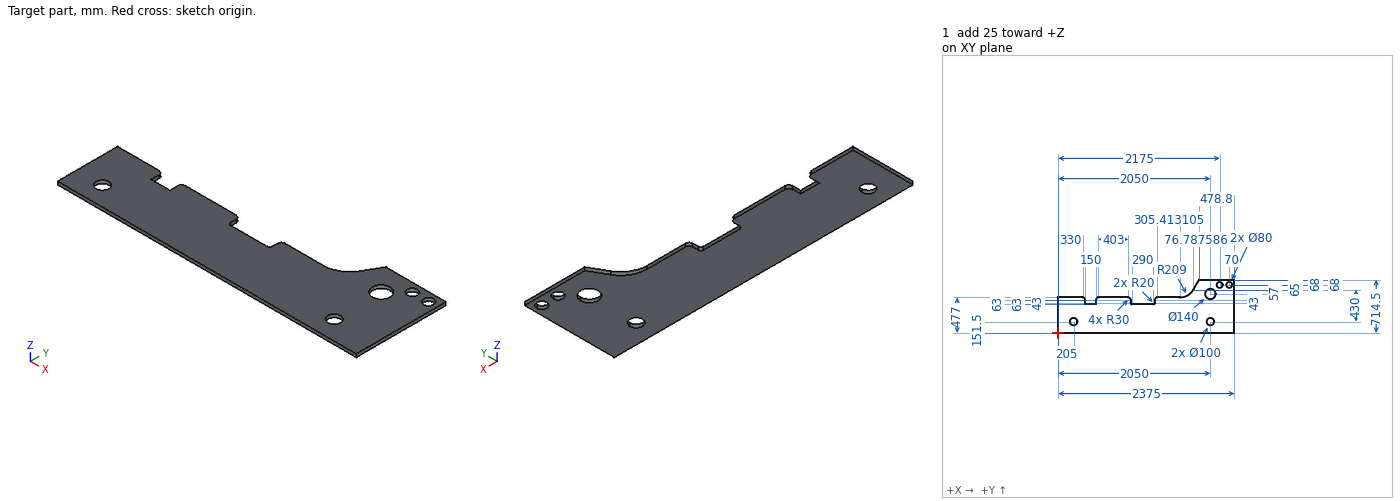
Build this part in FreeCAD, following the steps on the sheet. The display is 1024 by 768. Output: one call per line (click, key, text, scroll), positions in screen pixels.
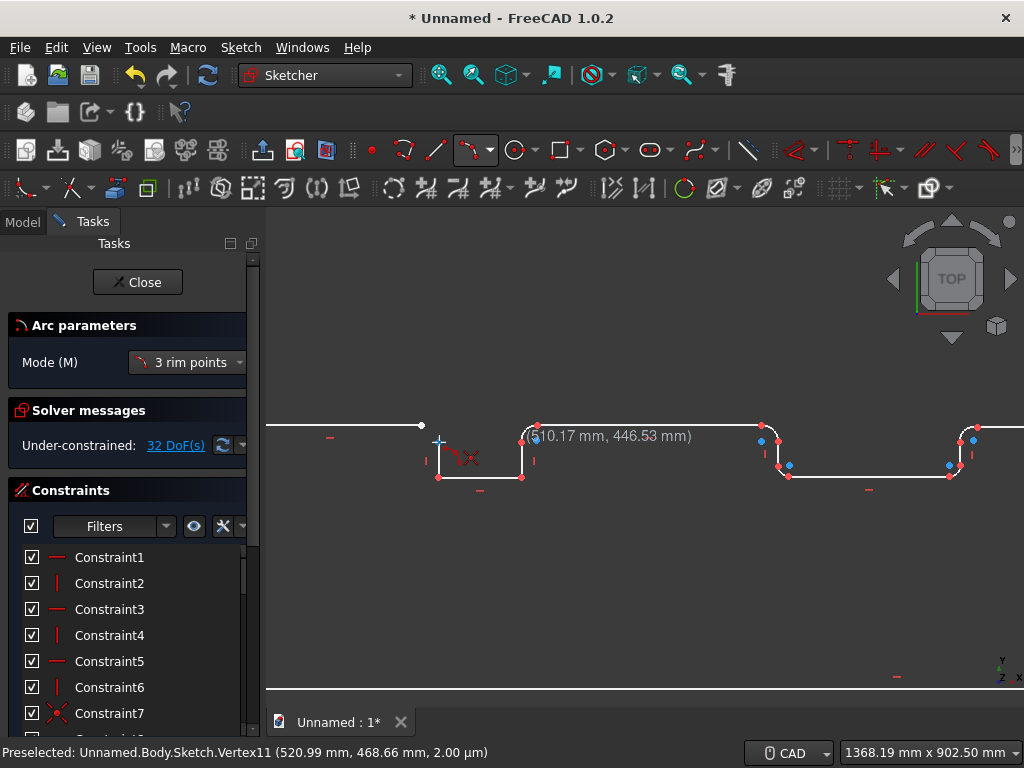
click(439, 442)
click(422, 425)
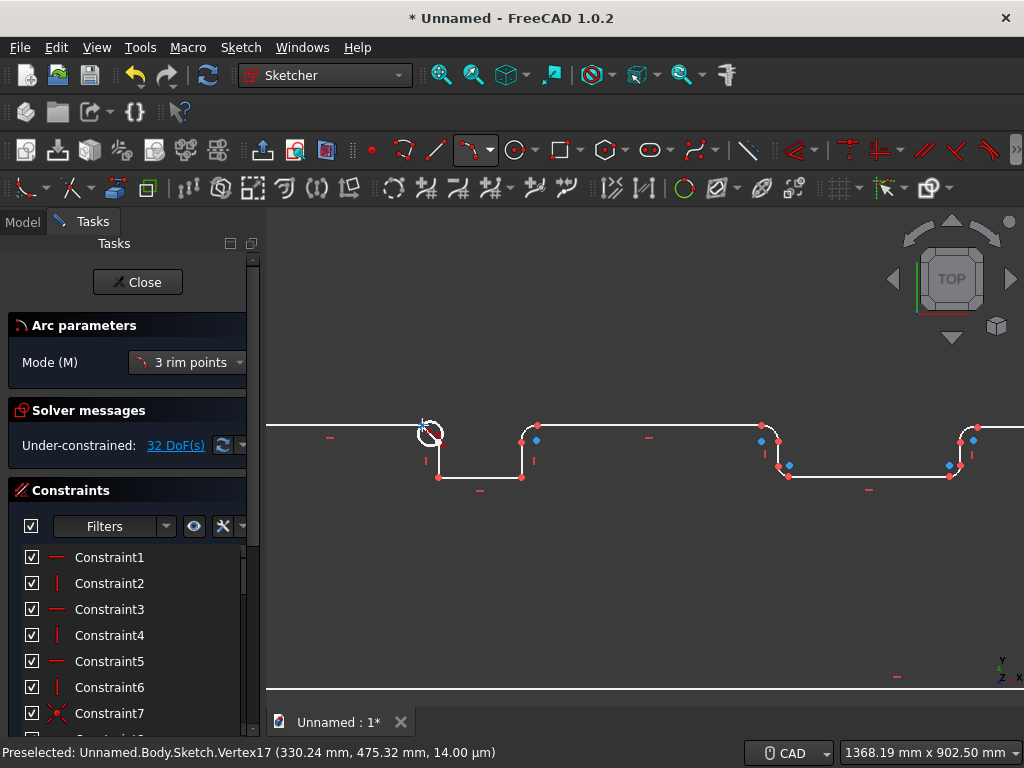
scroll(433, 429, up, 6)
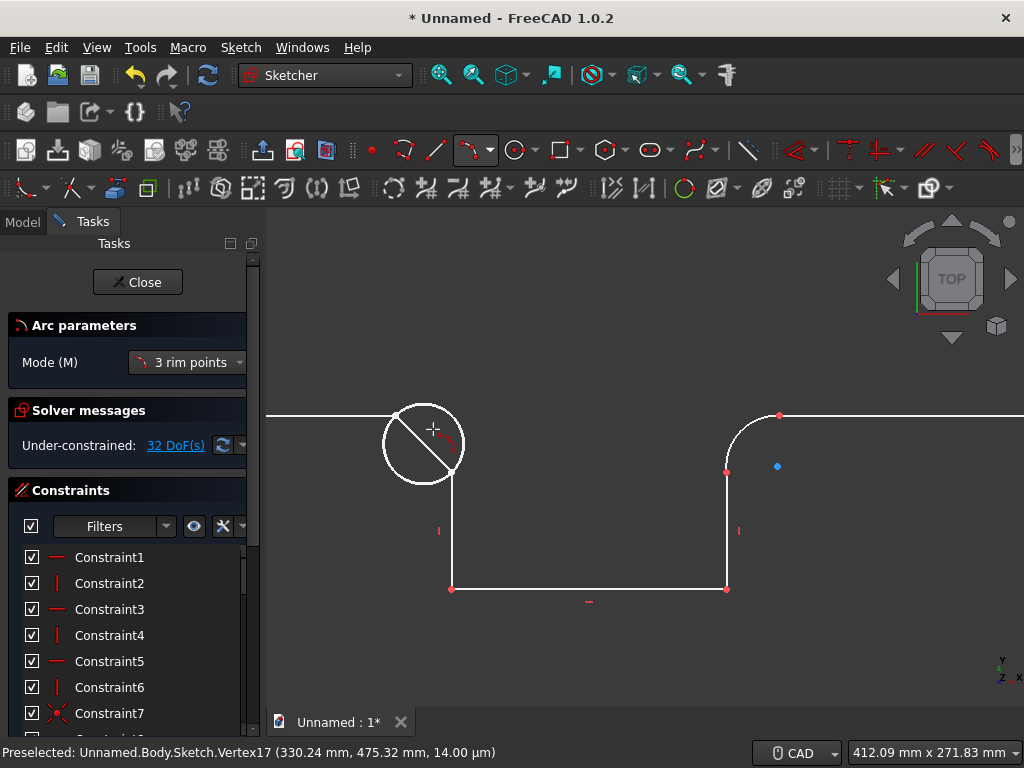
click(434, 429)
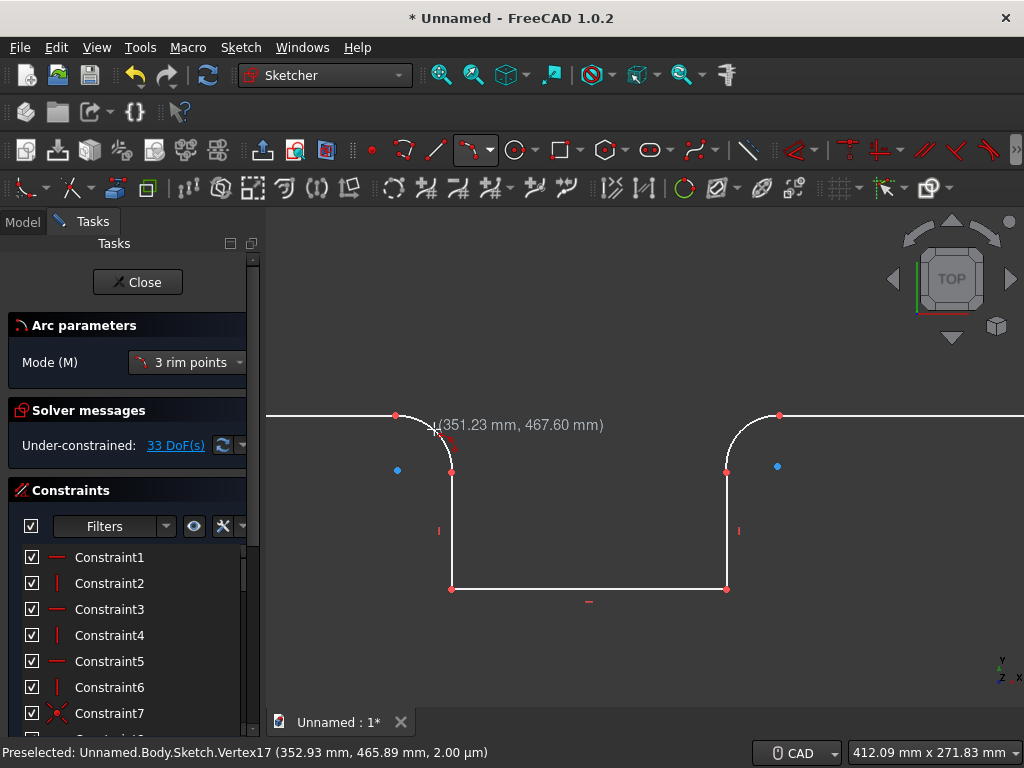
scroll(437, 439, down, 12)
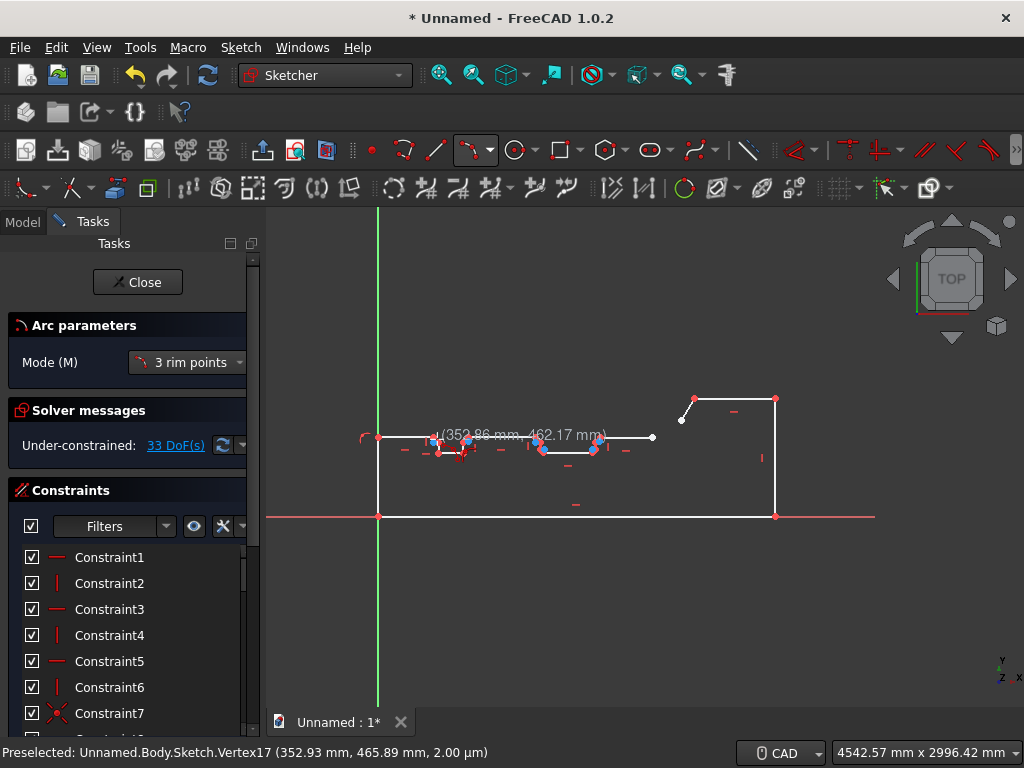
scroll(682, 420, up, 2)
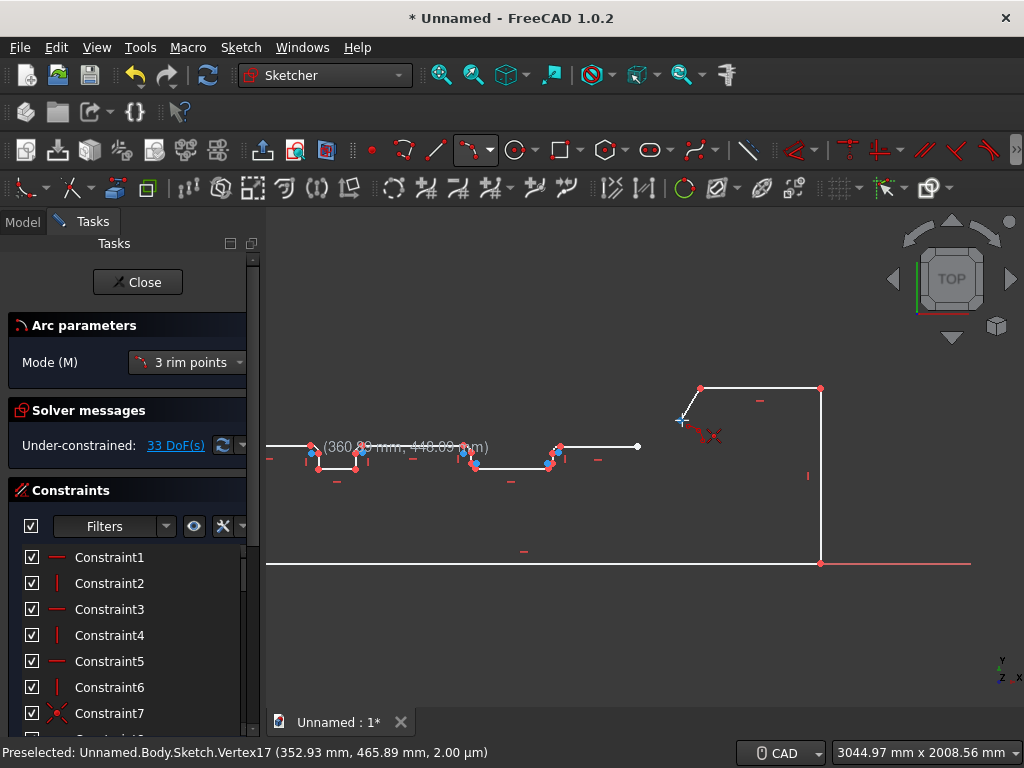
click(681, 421)
click(637, 447)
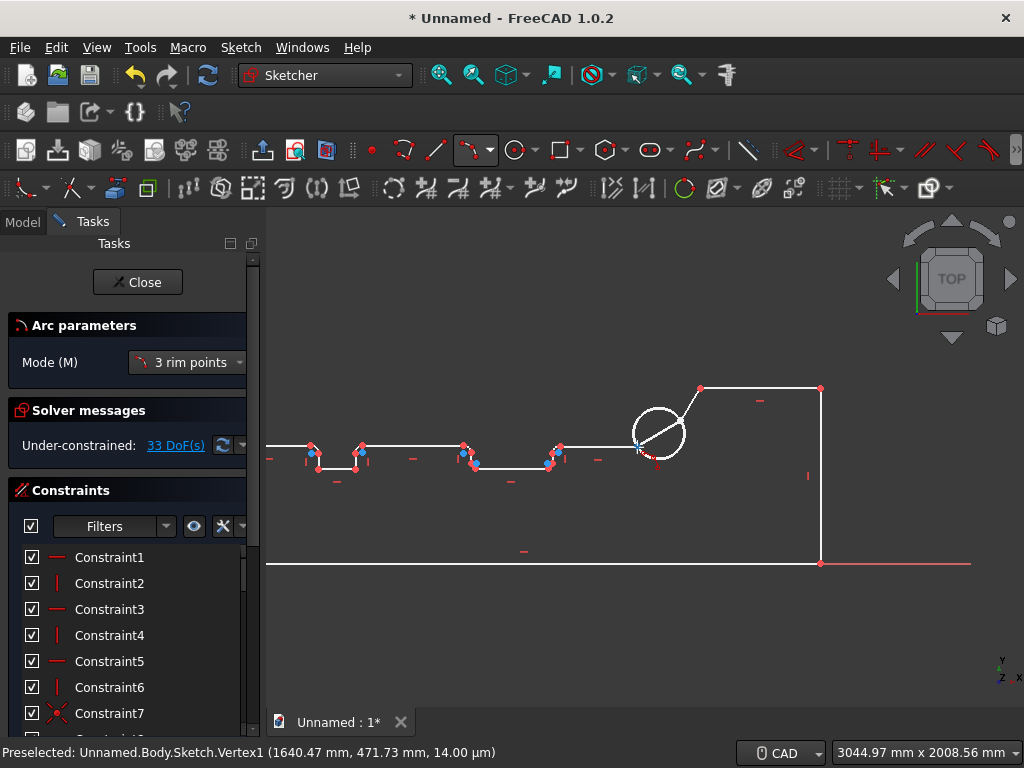
scroll(663, 438, up, 5)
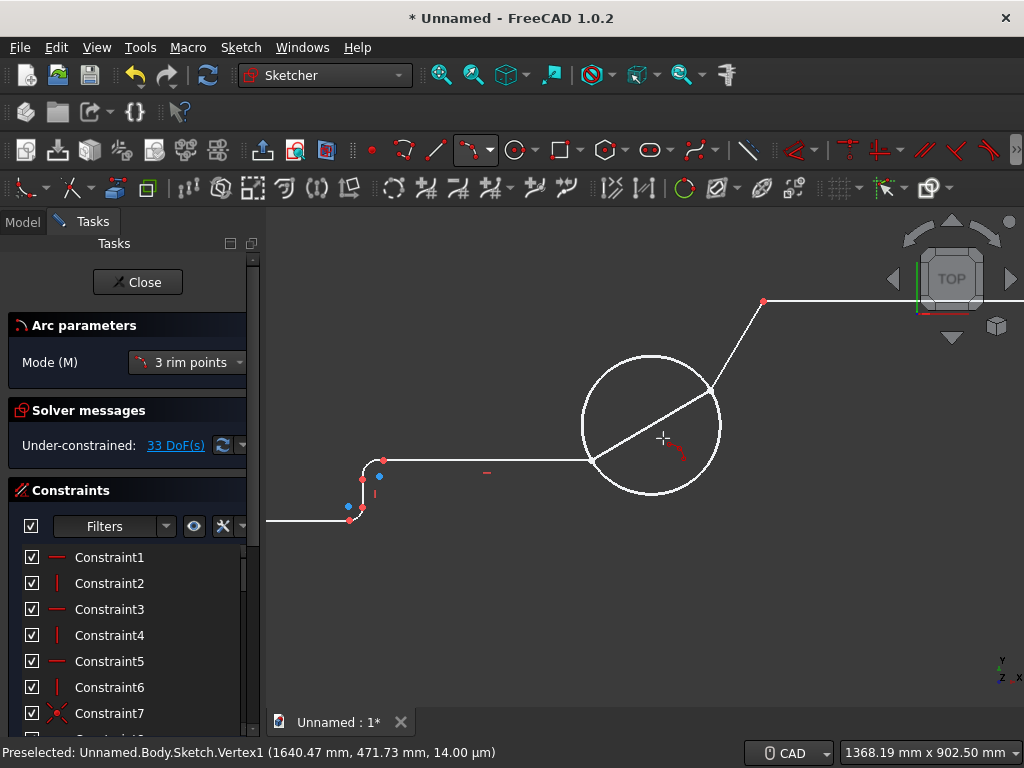
click(661, 438)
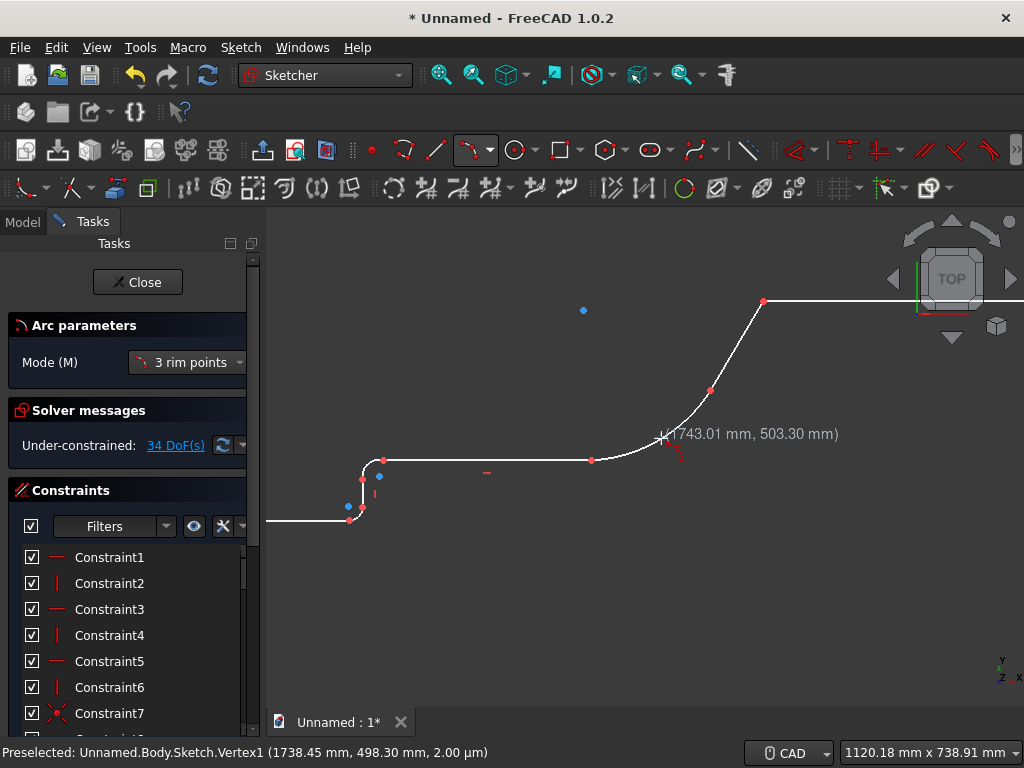
click(516, 150)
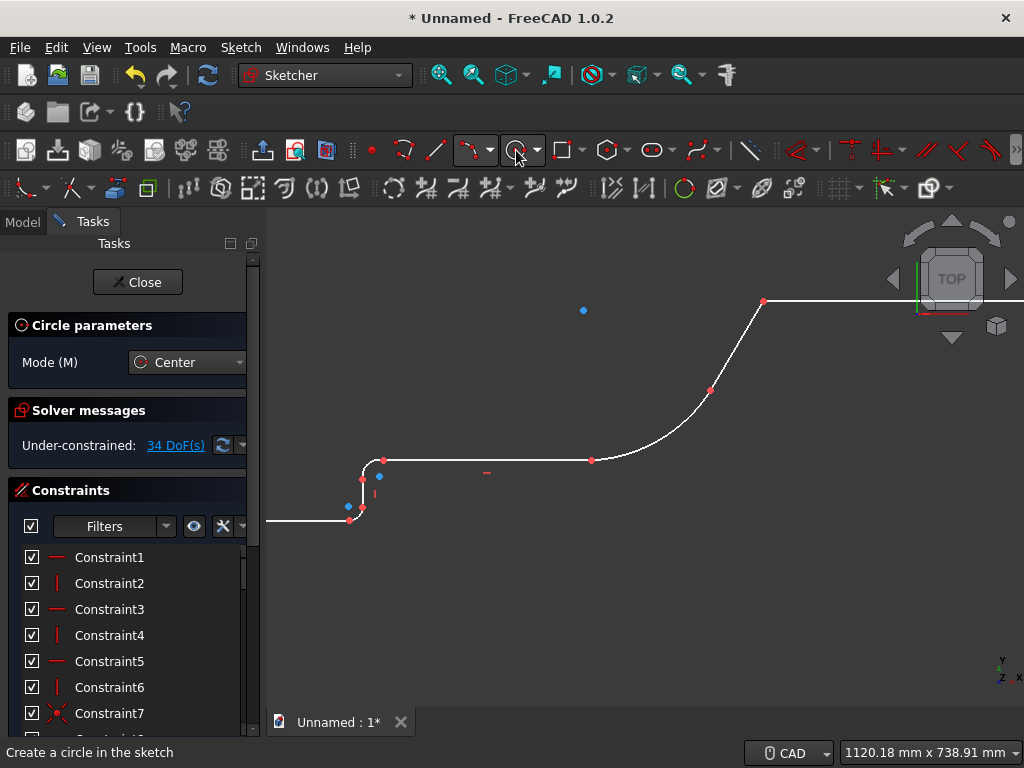
scroll(672, 431, down, 7)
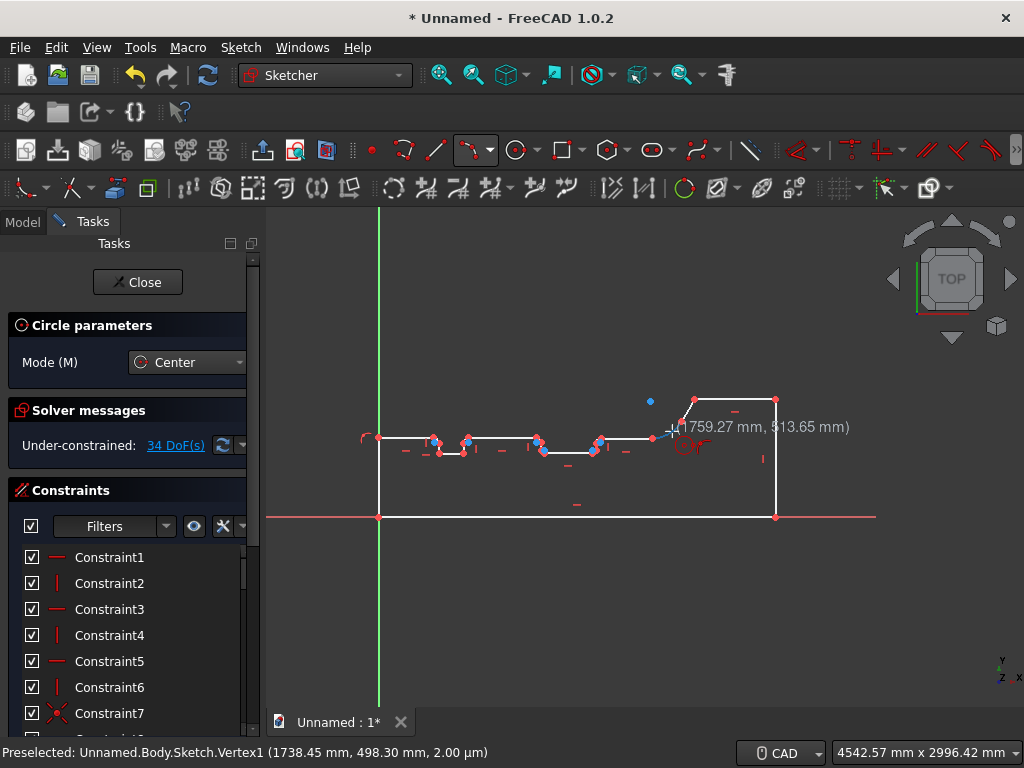
scroll(721, 492, up, 6)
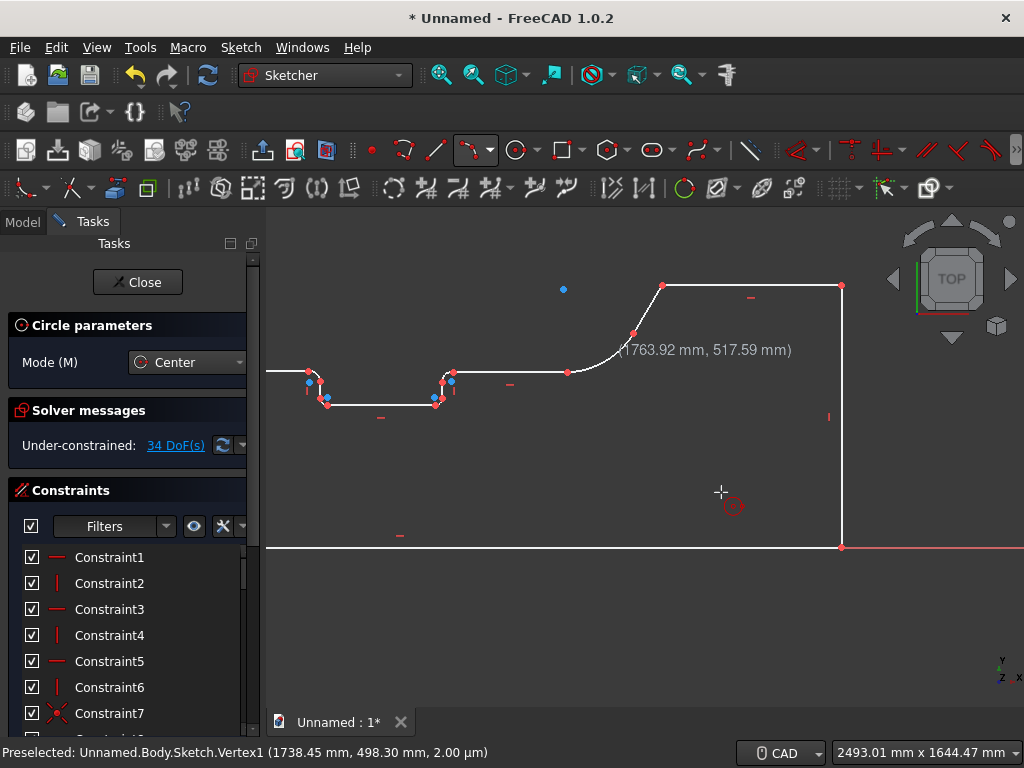
click(719, 491)
move(739, 471)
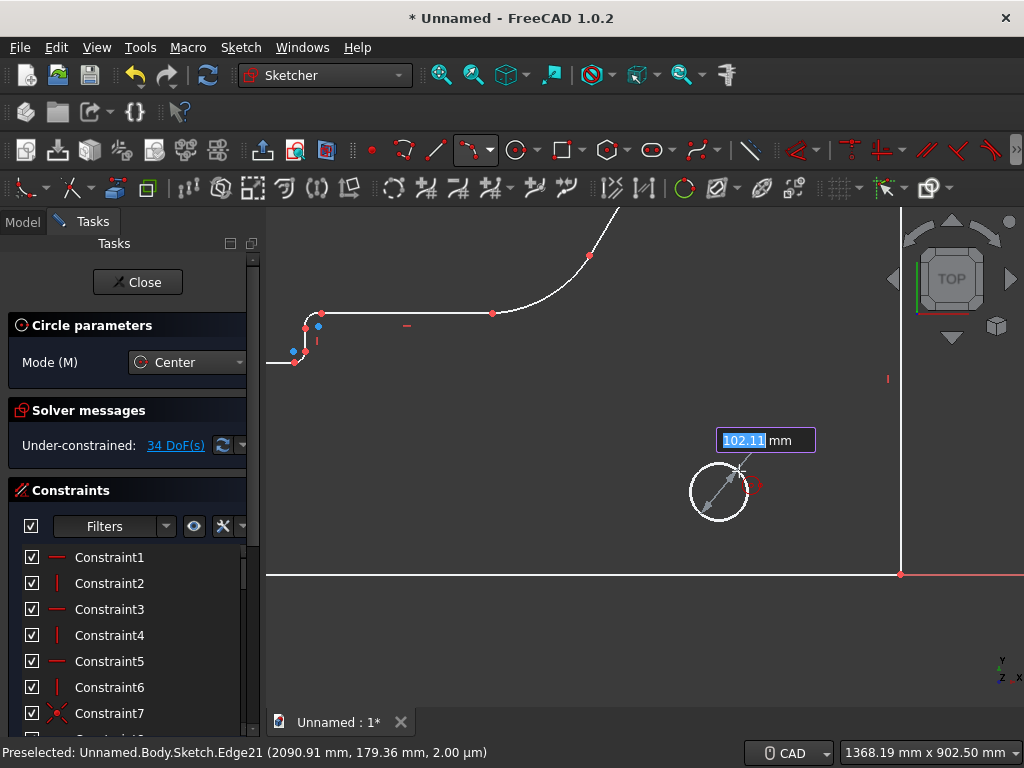
text(100)
key(Return)